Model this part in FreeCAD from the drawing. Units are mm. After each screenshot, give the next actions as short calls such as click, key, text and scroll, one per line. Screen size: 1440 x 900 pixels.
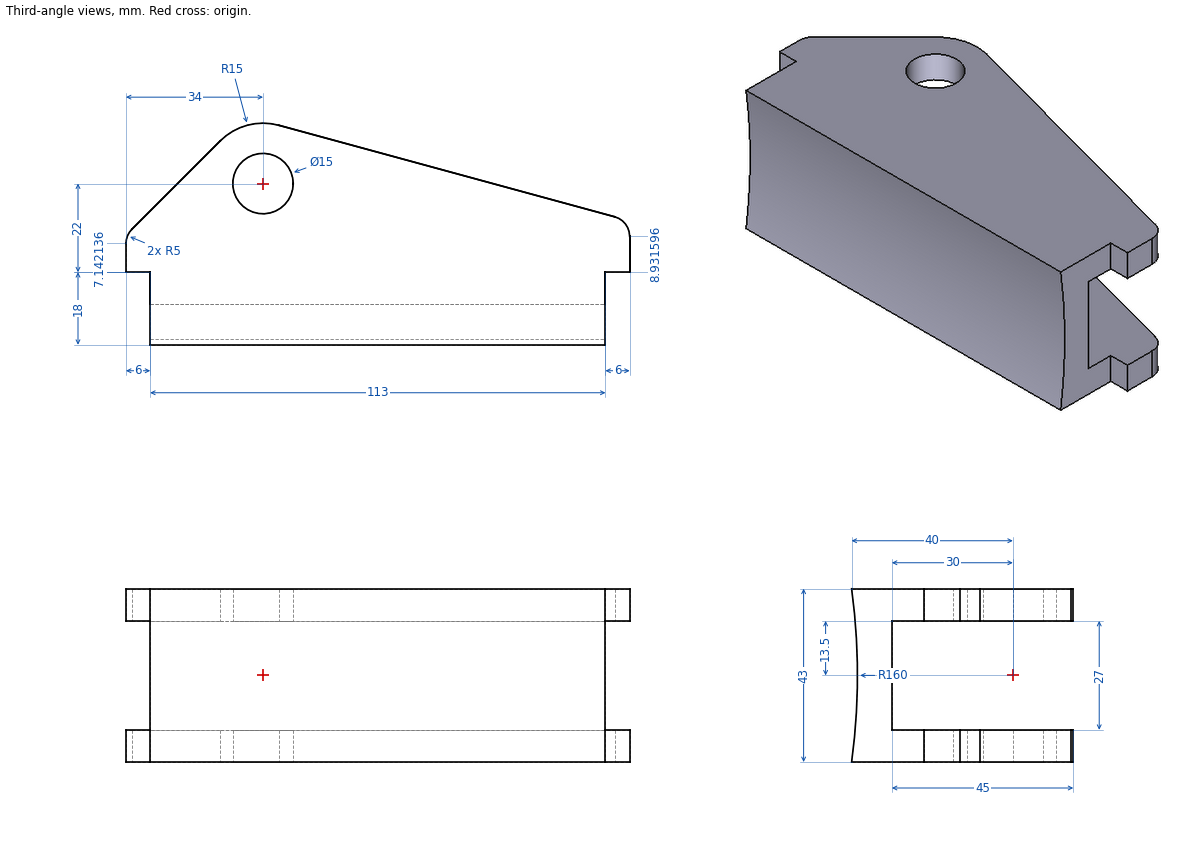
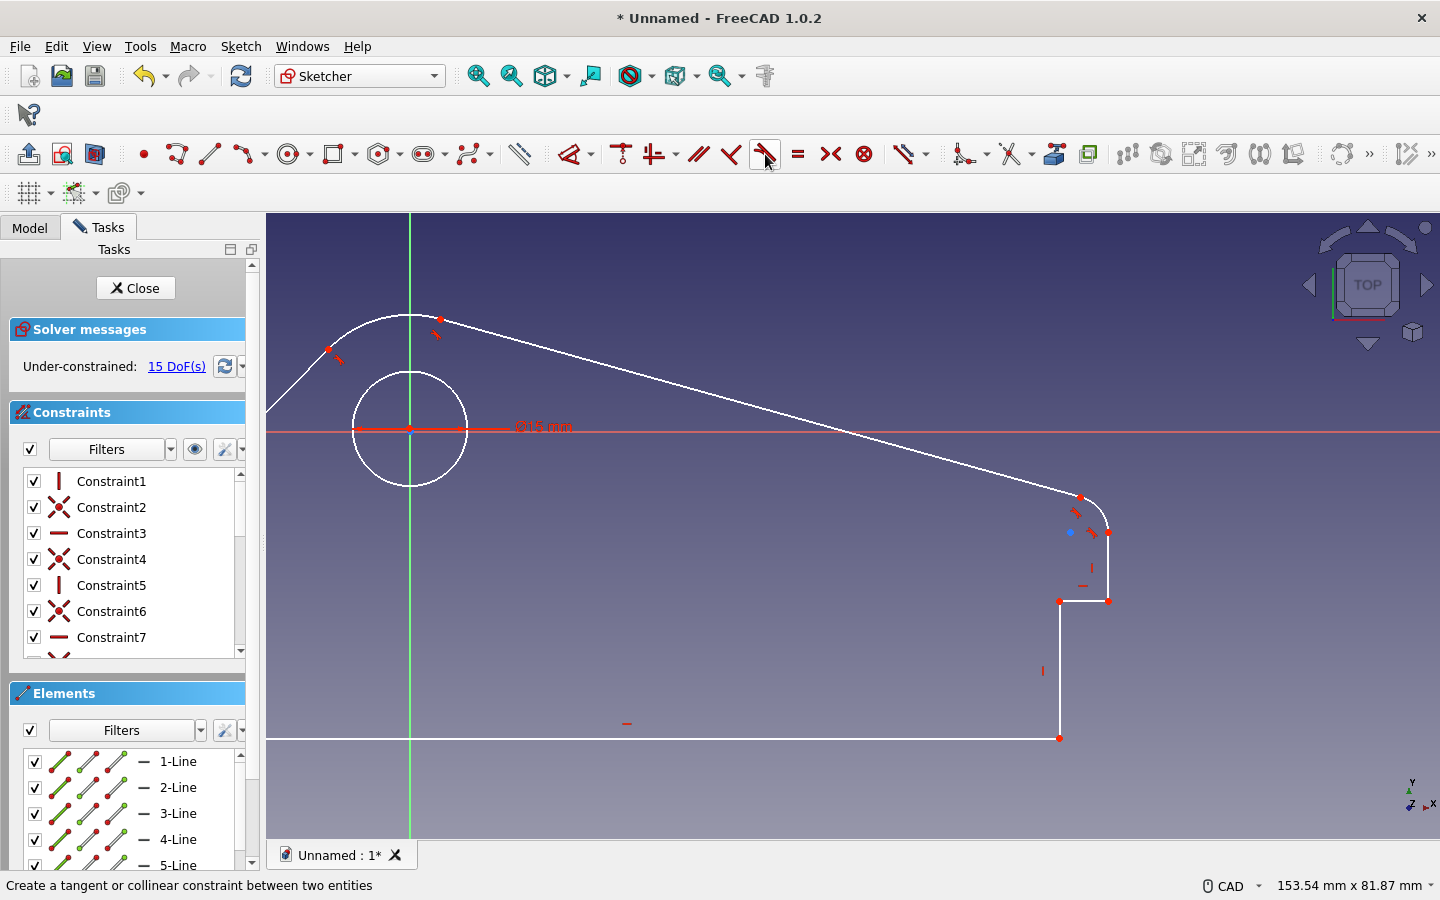
click(295, 383)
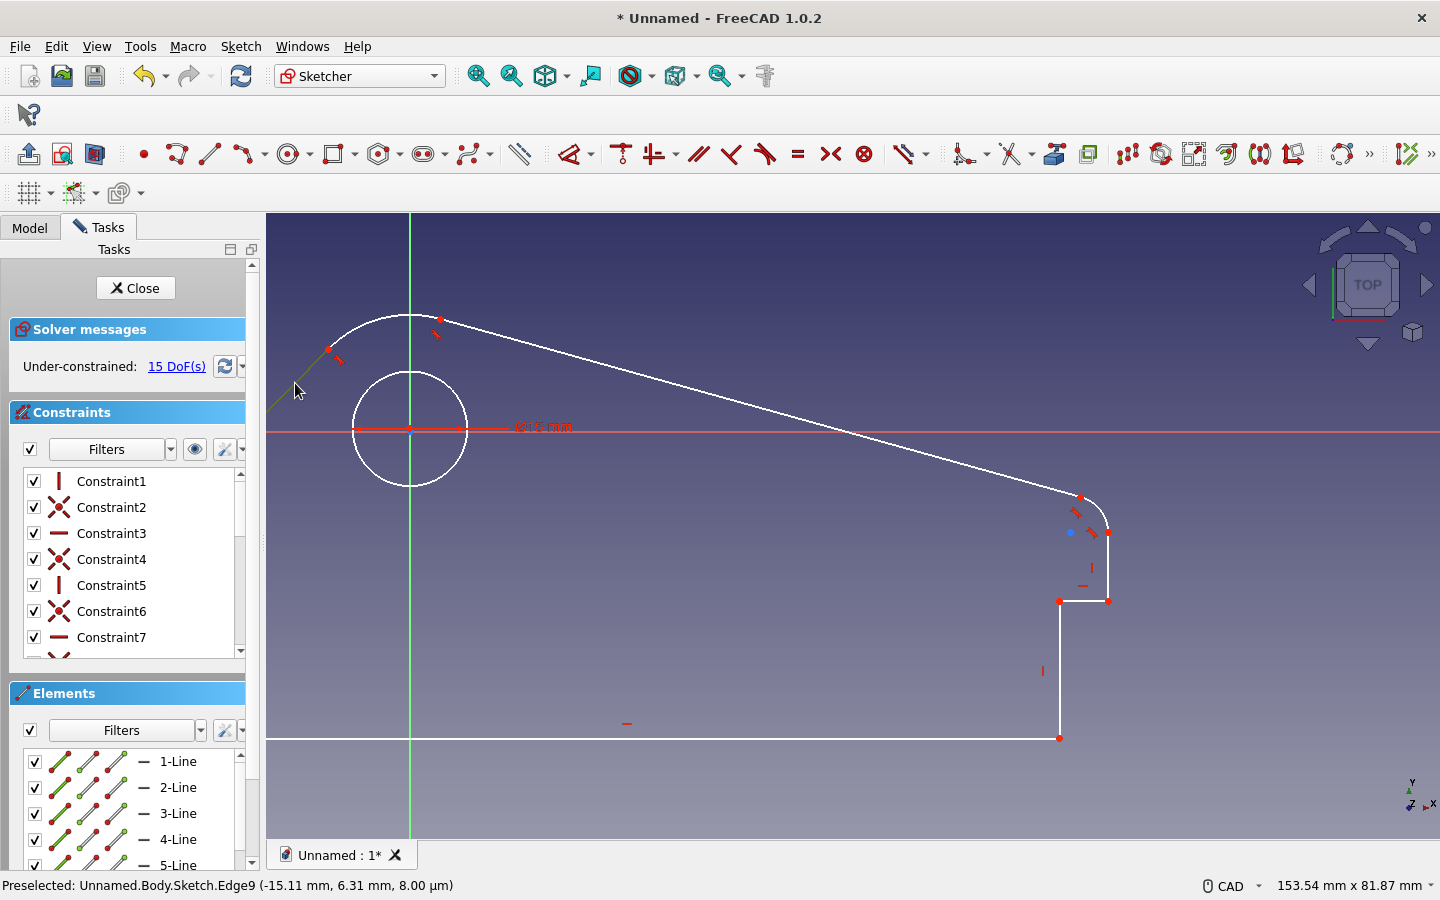
scroll(1103, 519, down, 2)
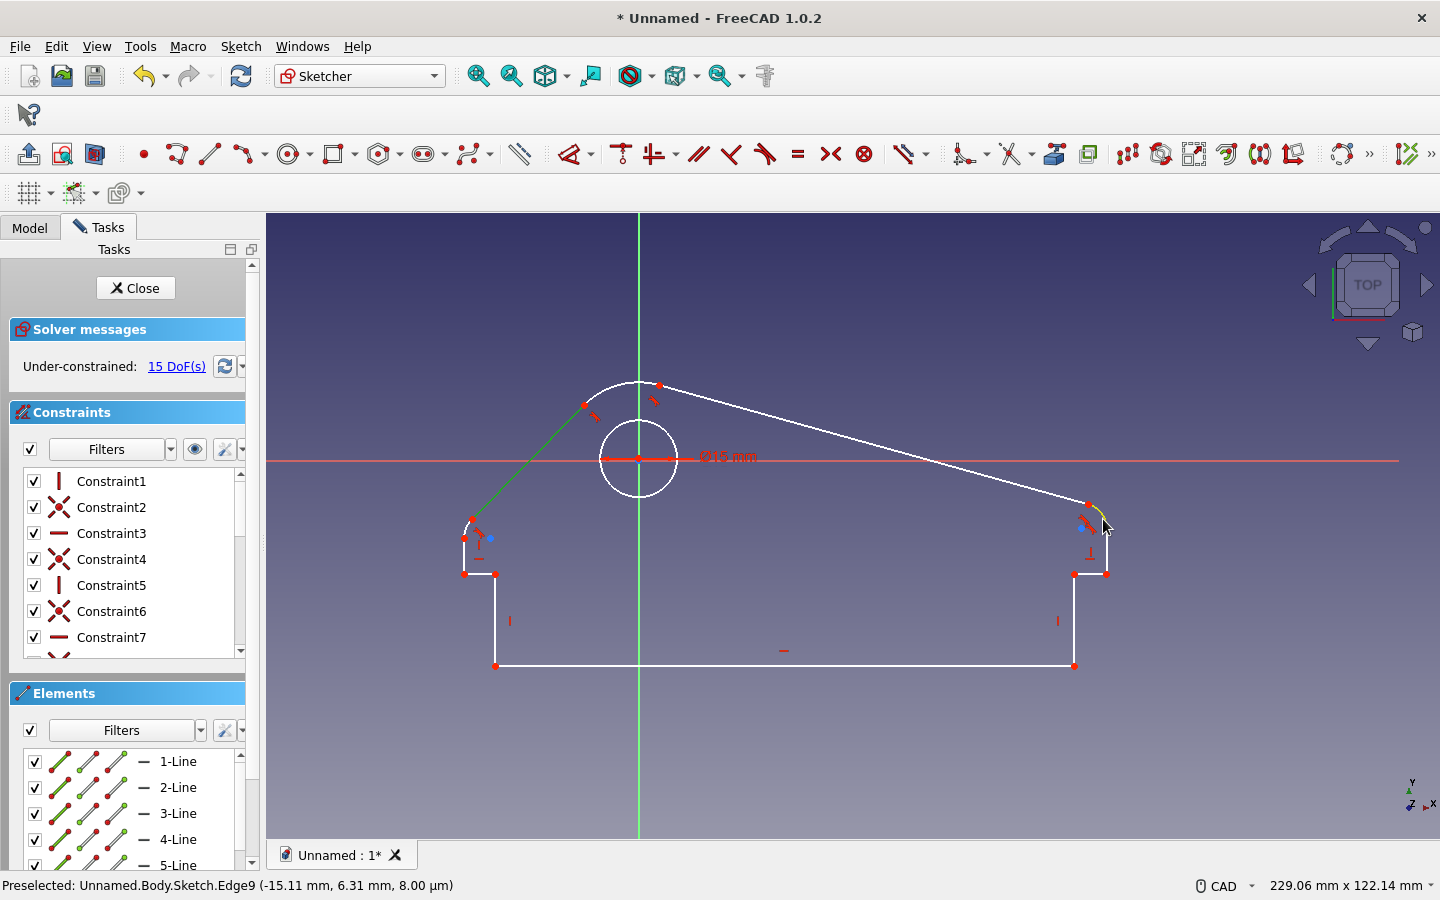
scroll(468, 524, up, 4)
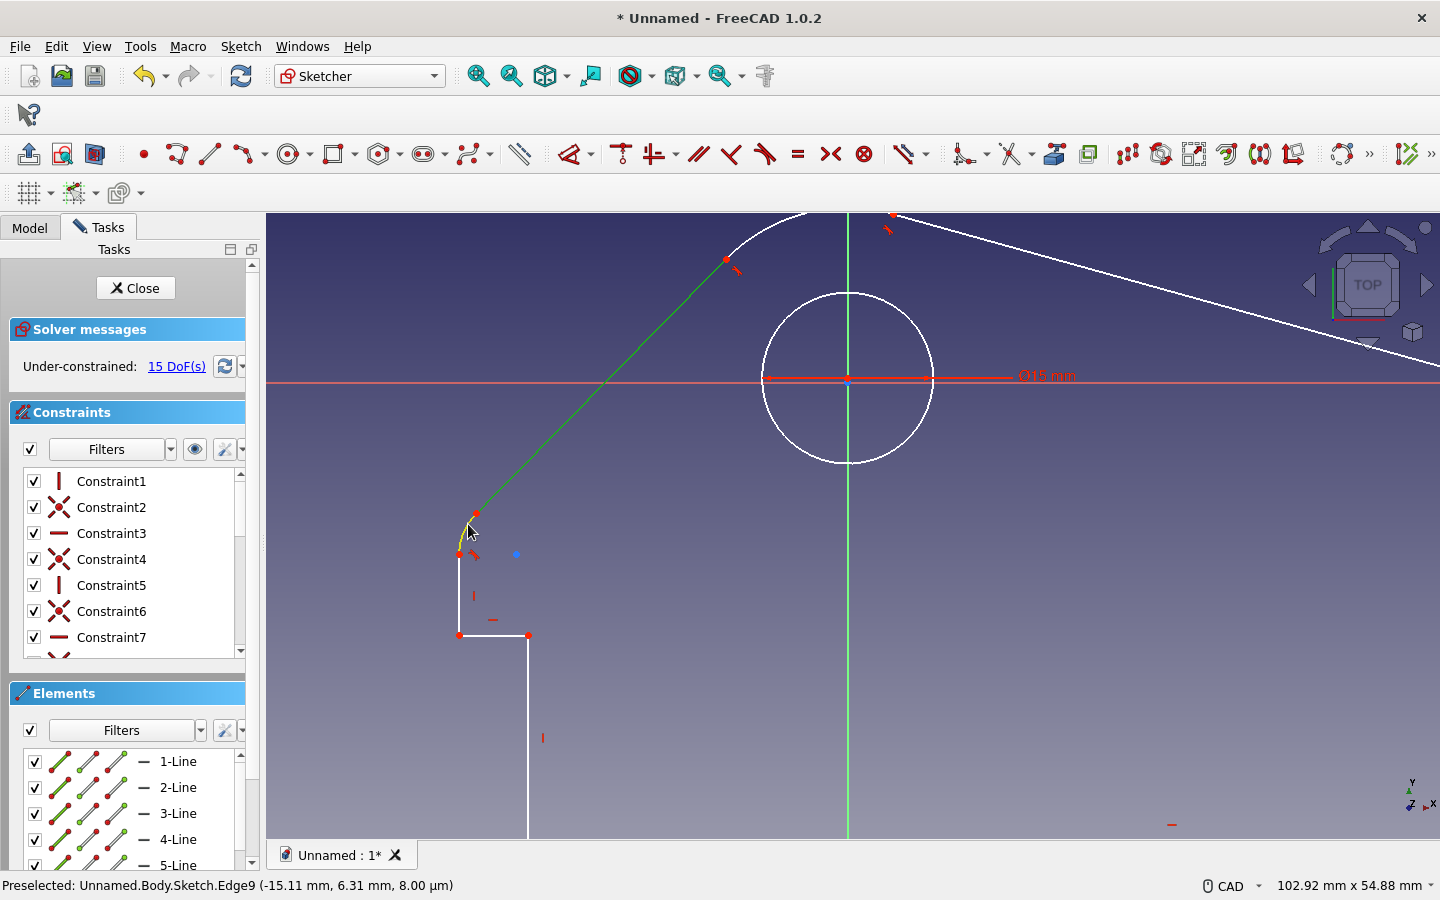
click(468, 524)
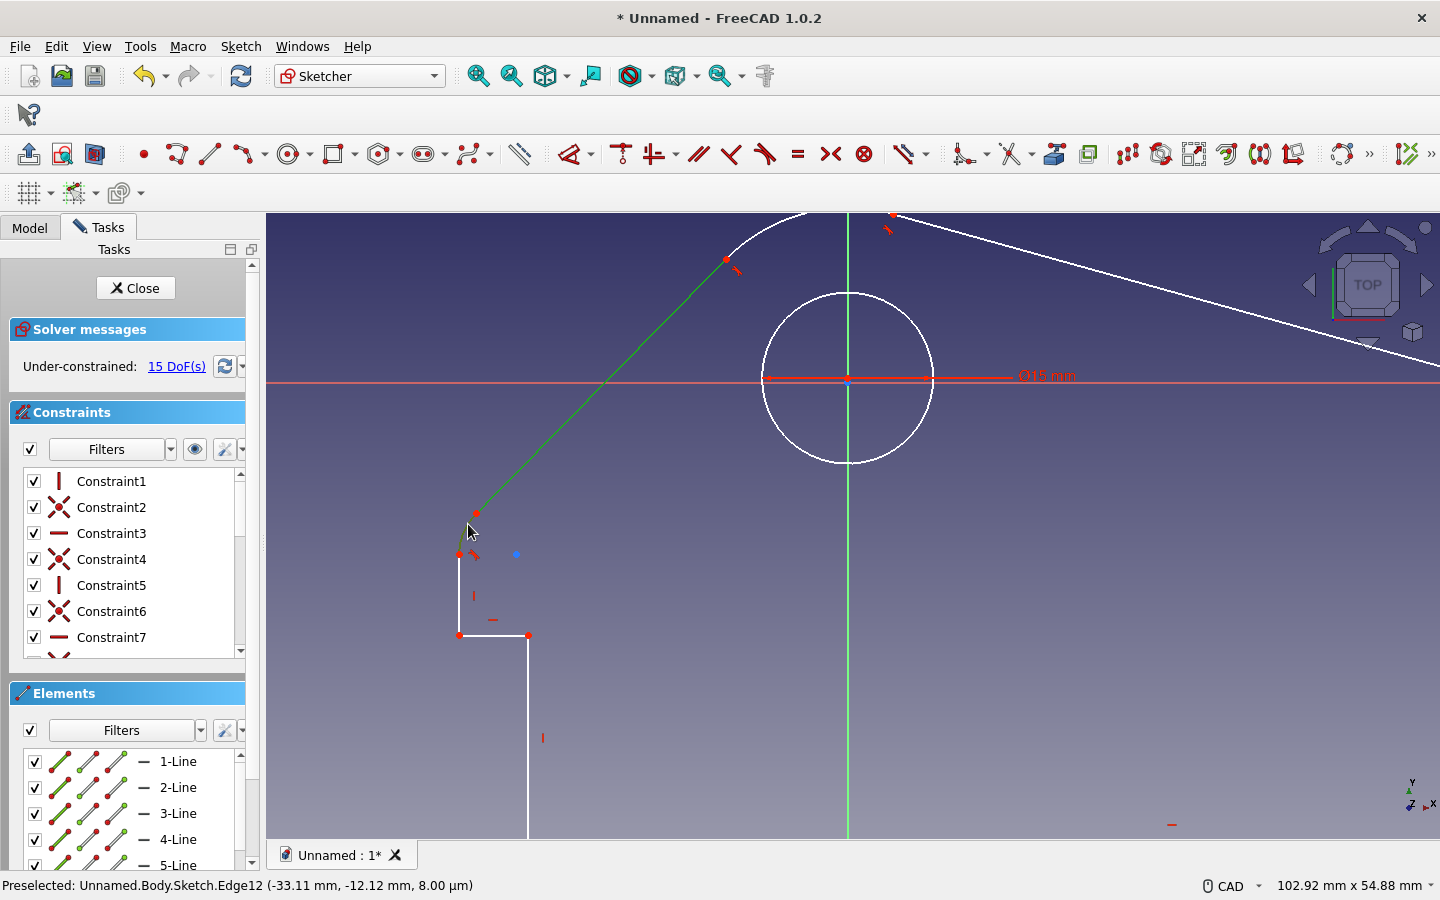
click(765, 154)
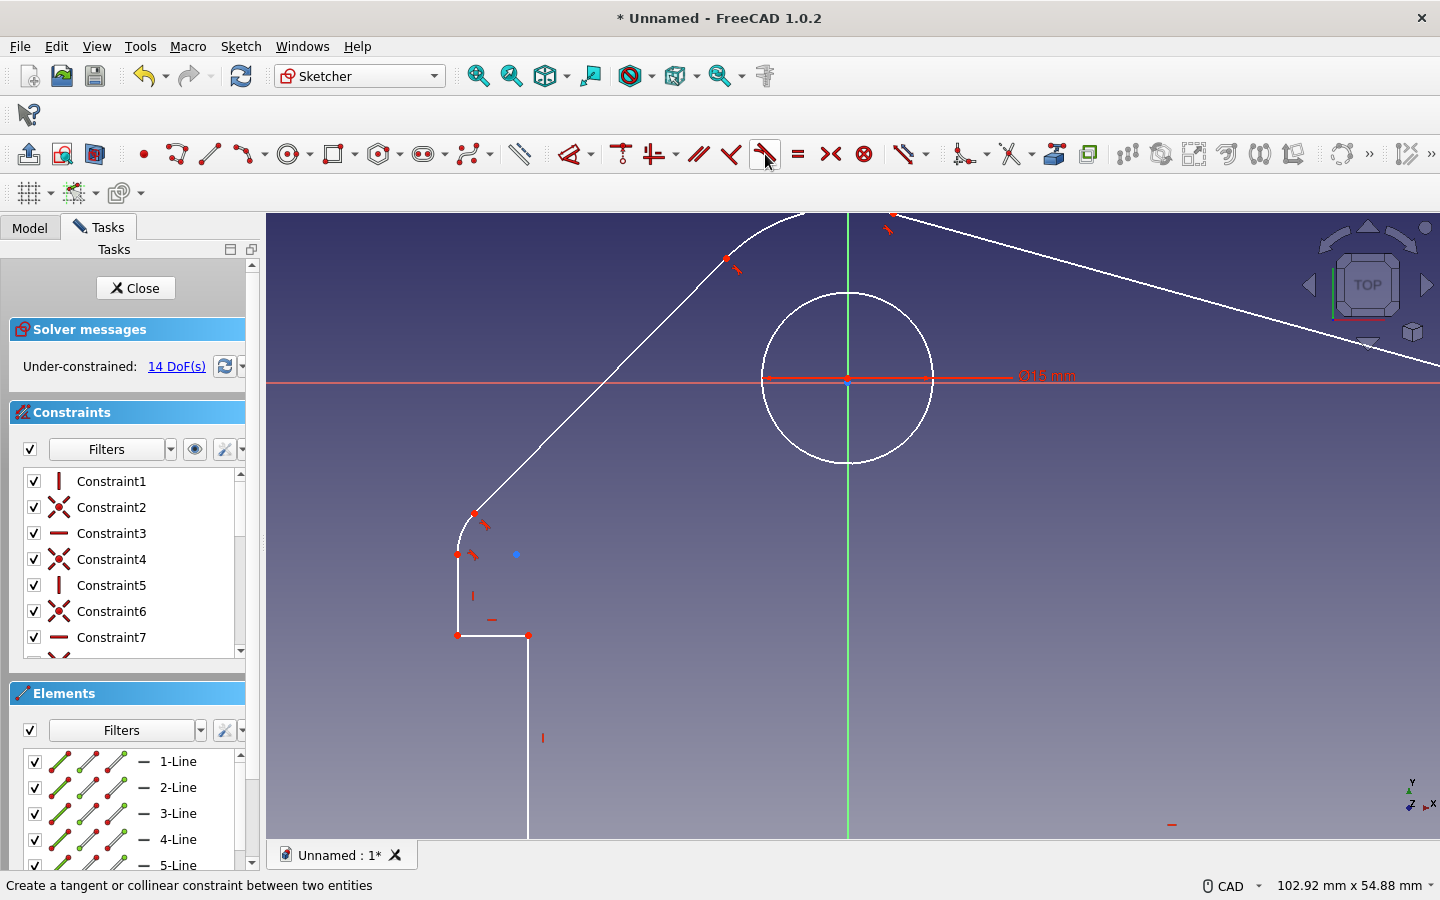
drag(837, 368, 858, 393)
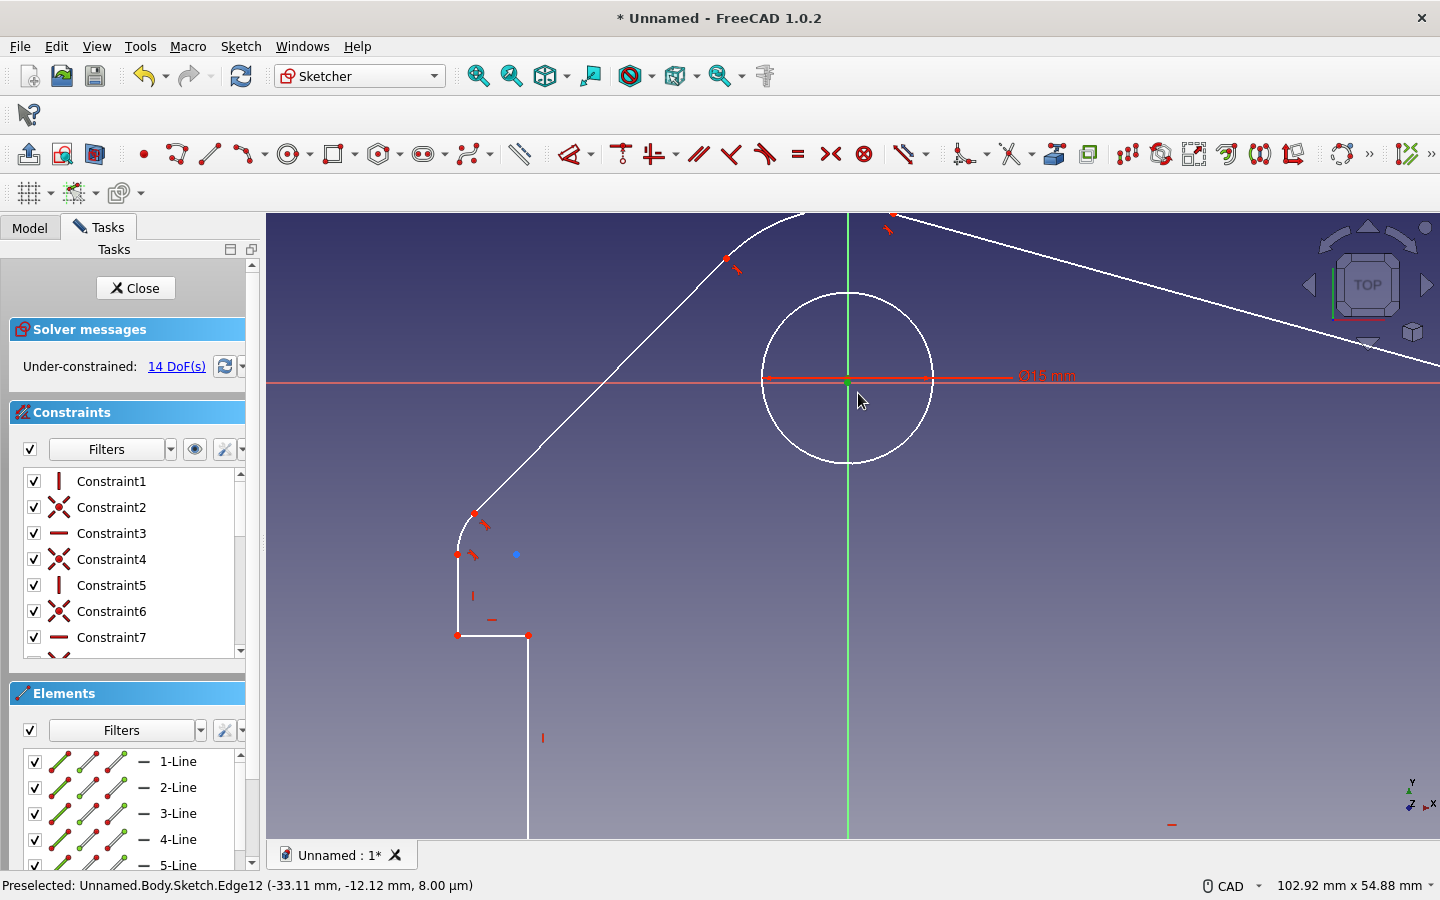
click(621, 154)